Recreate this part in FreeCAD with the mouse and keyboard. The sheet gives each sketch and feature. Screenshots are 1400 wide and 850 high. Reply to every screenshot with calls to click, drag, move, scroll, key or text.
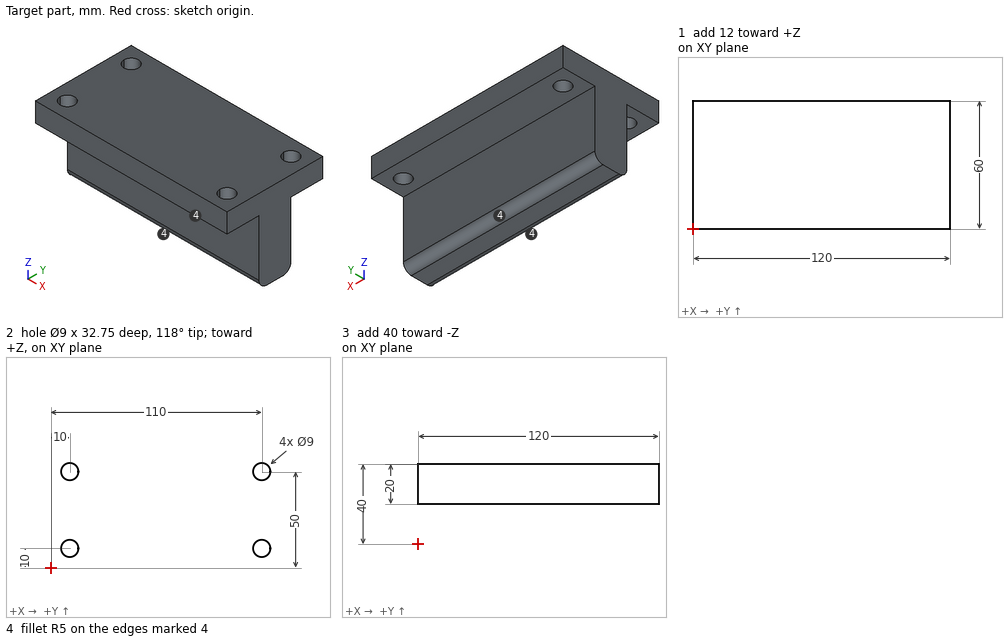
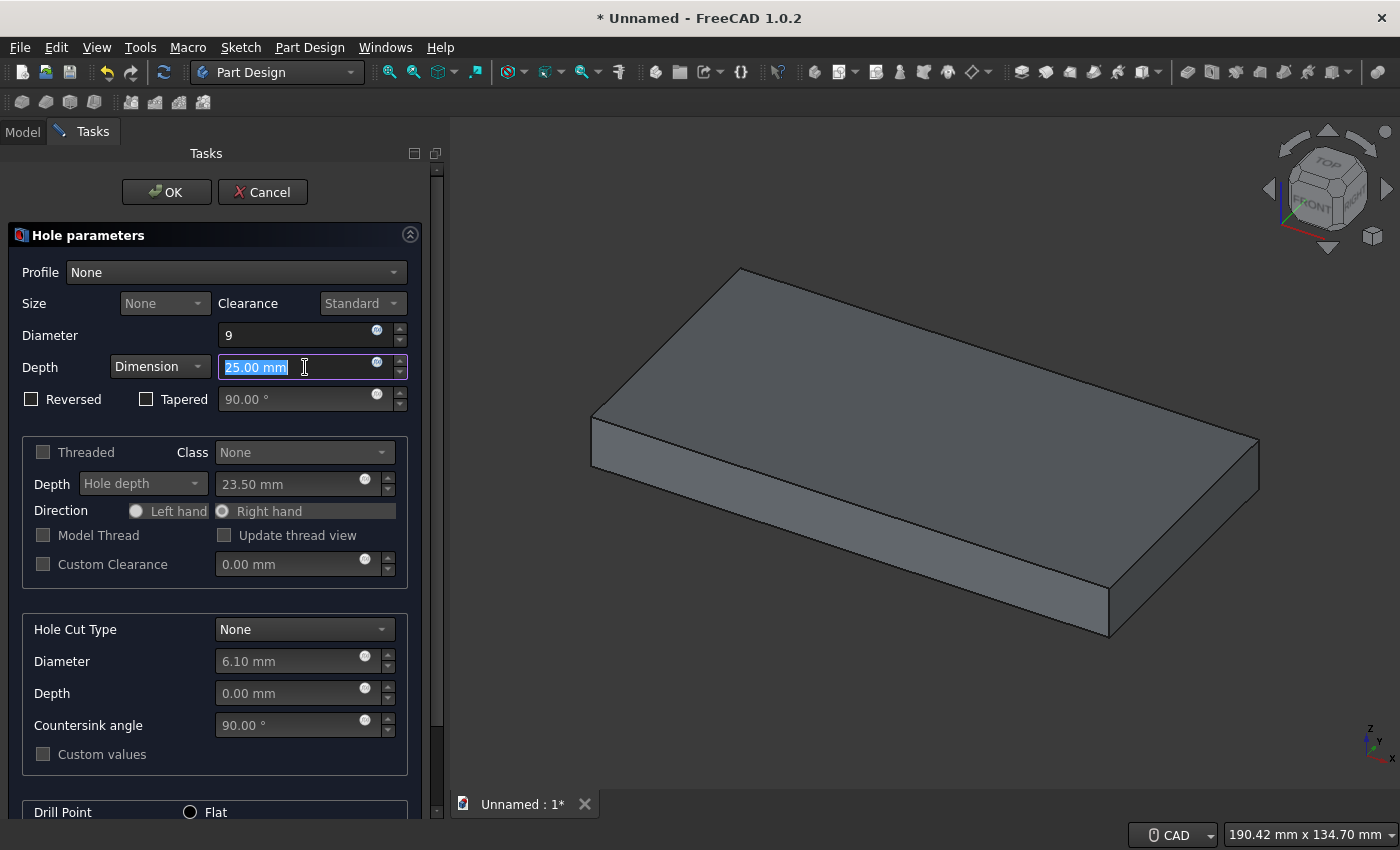
text(32.75)
key(Tab)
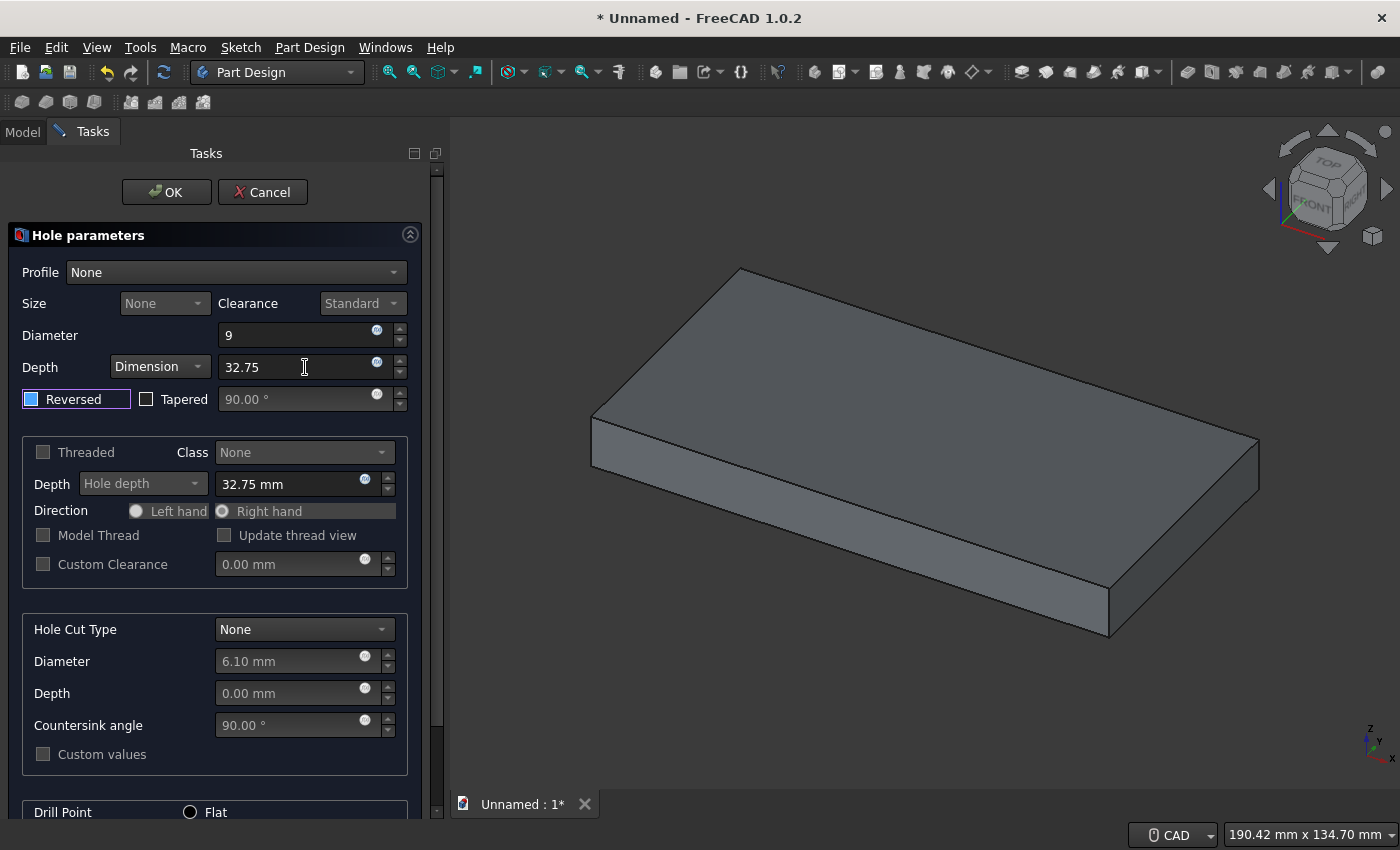
click(30, 399)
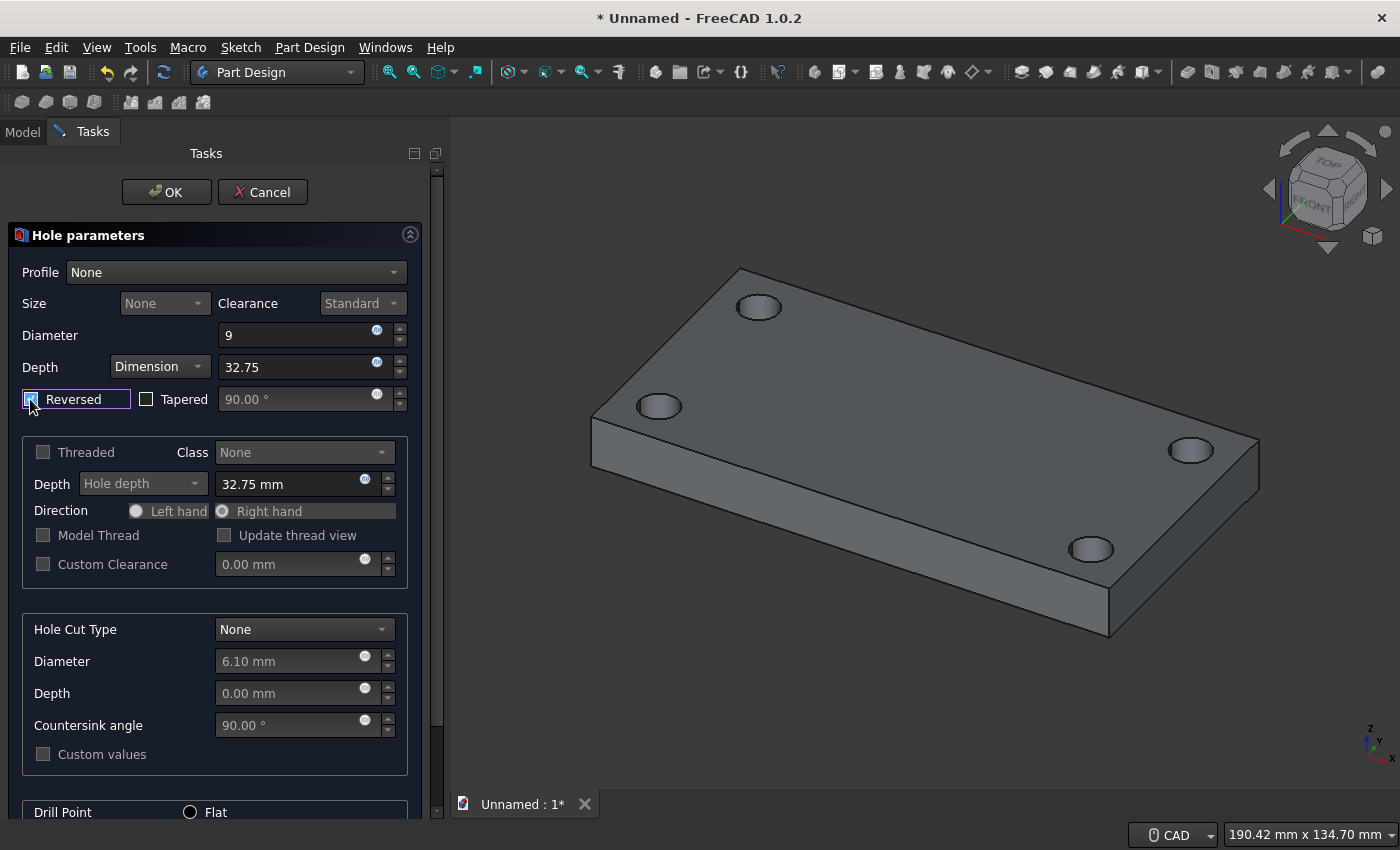
click(167, 192)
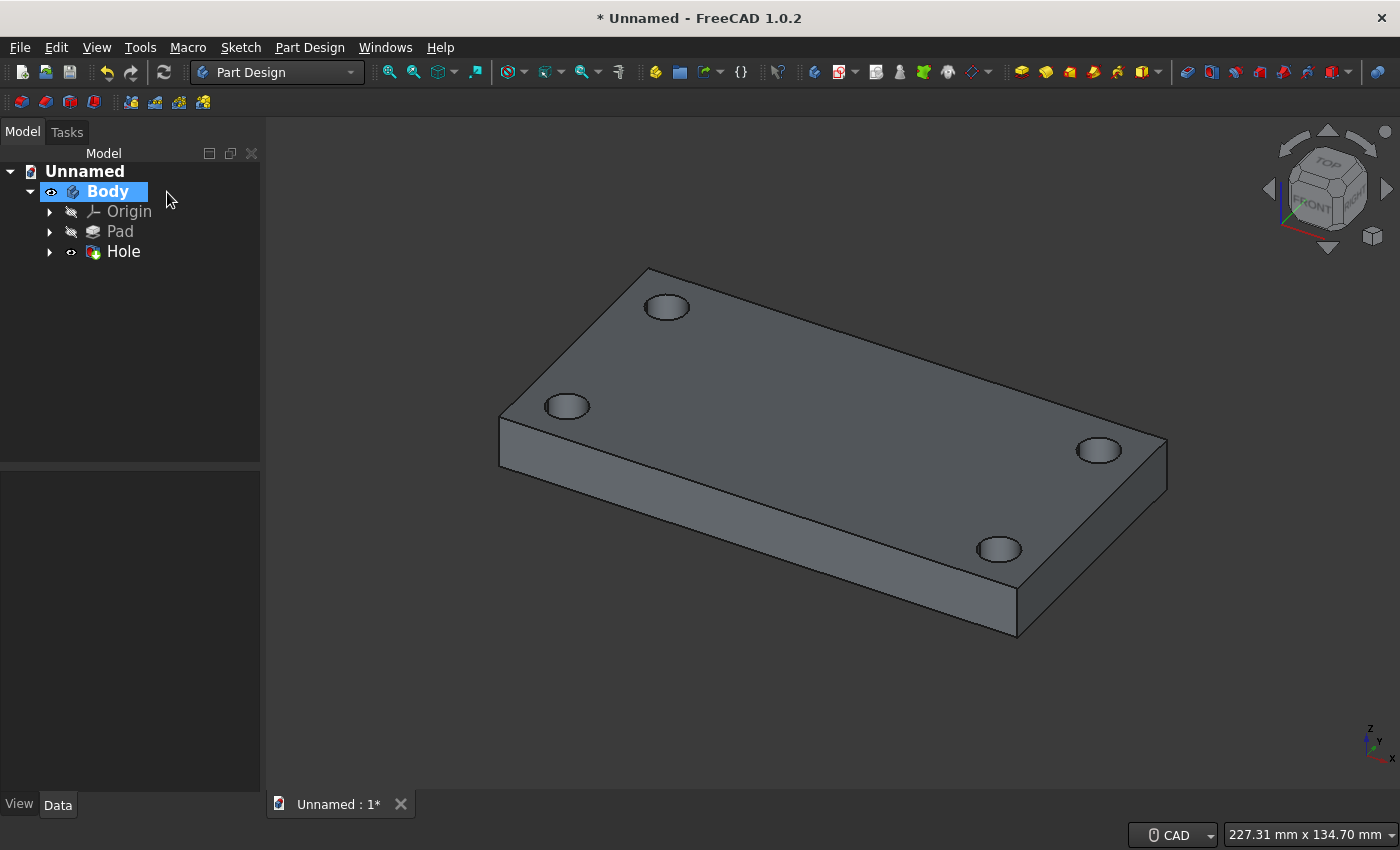
click(840, 72)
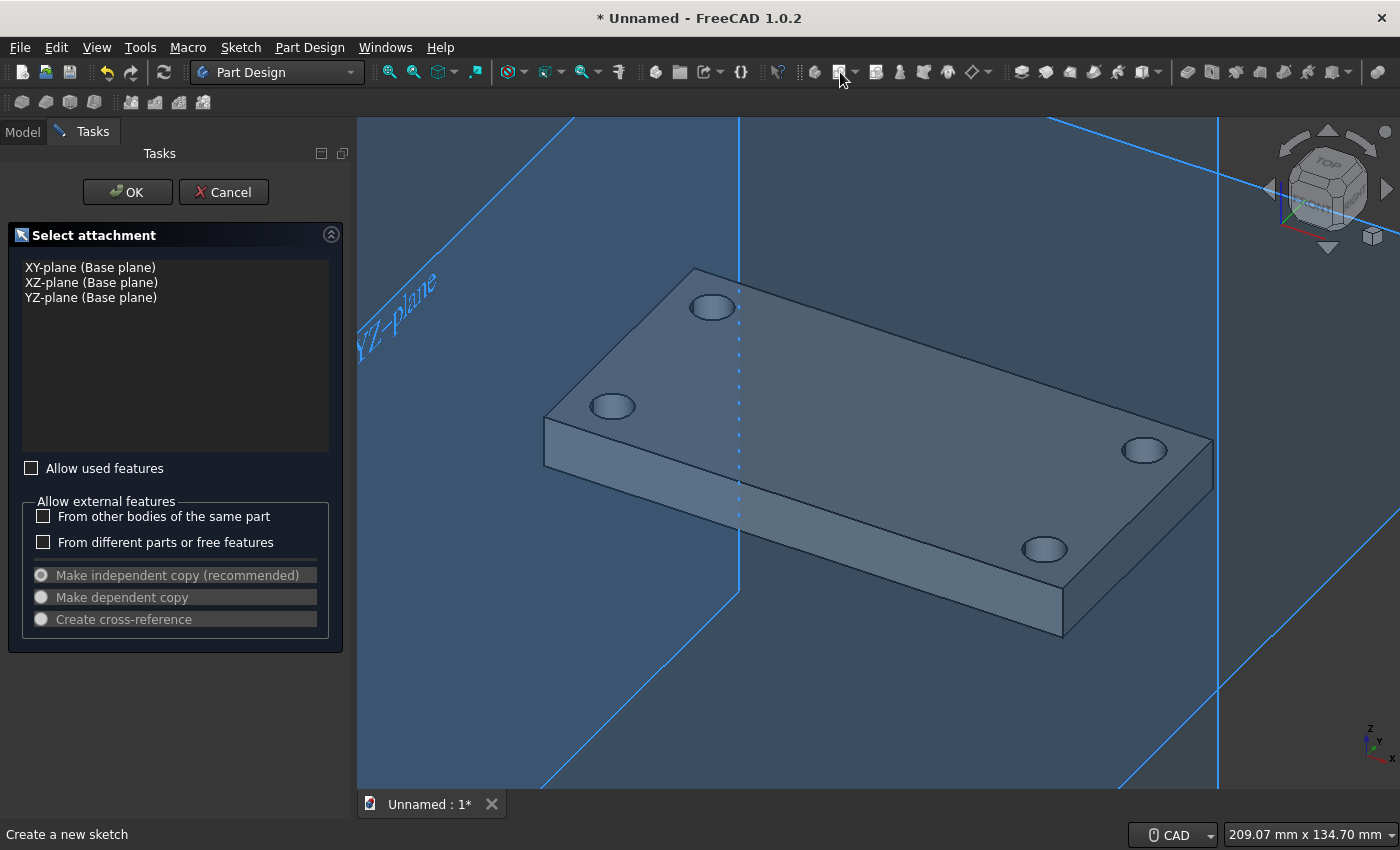
click(82, 268)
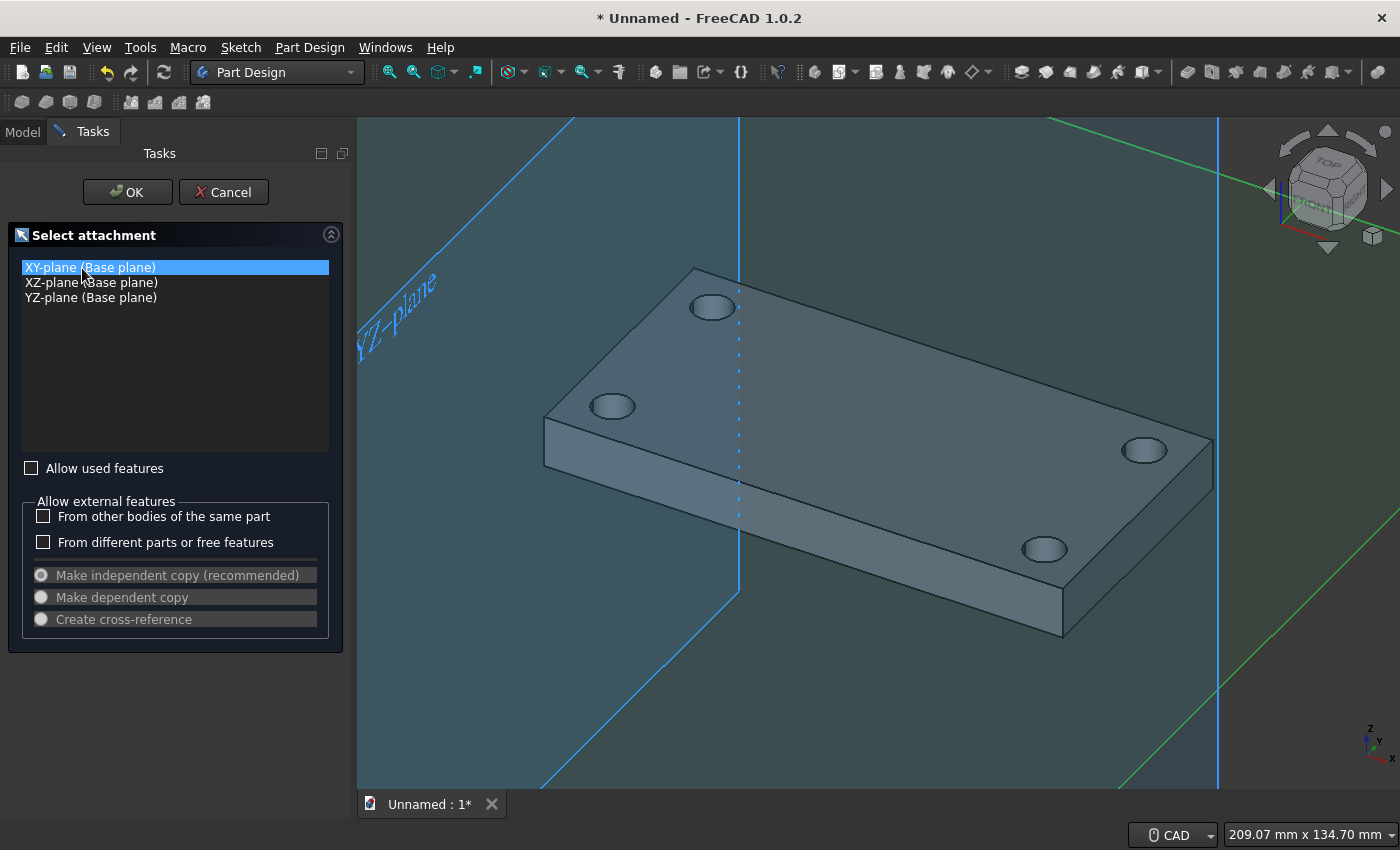
click(128, 192)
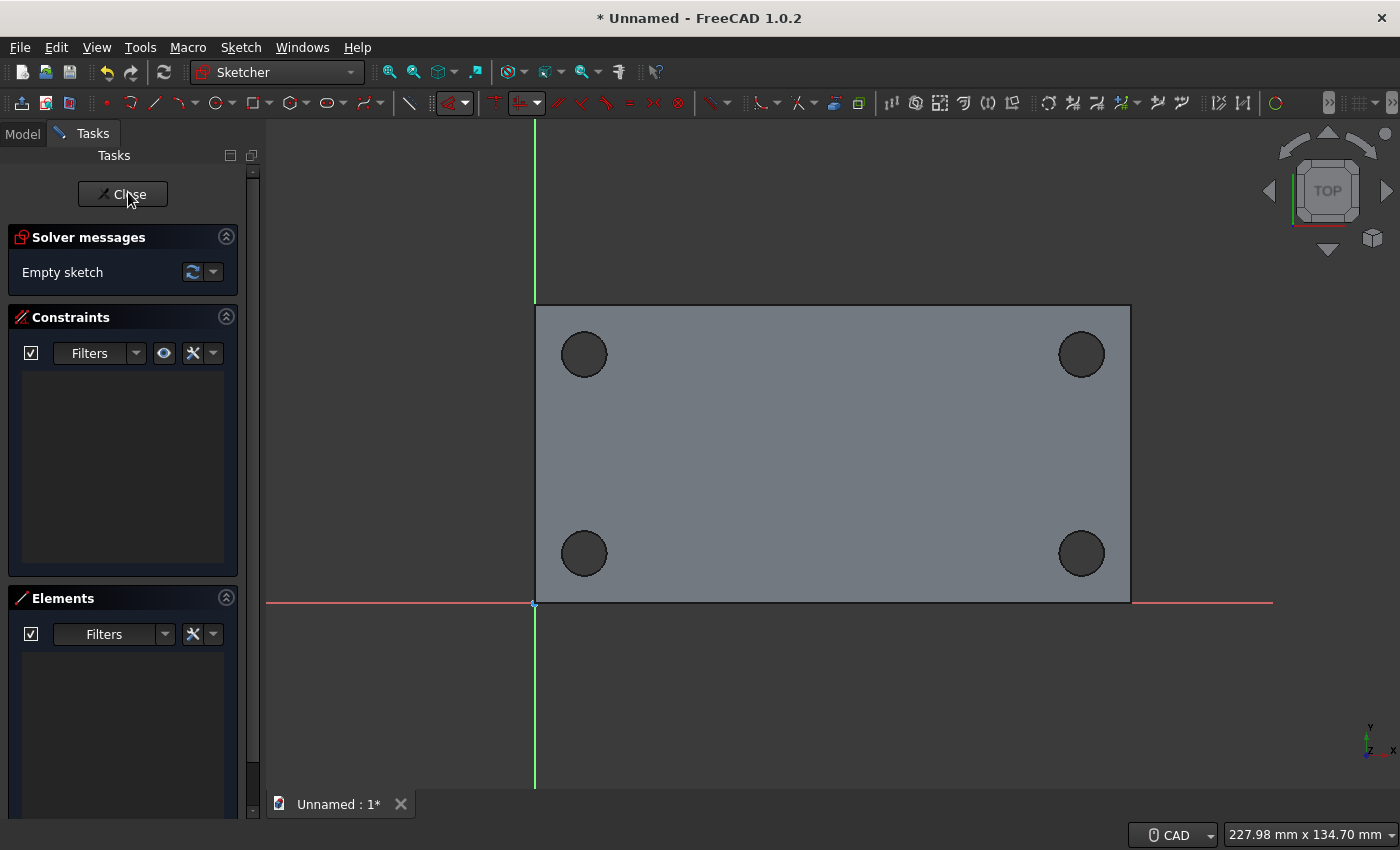
click(70, 104)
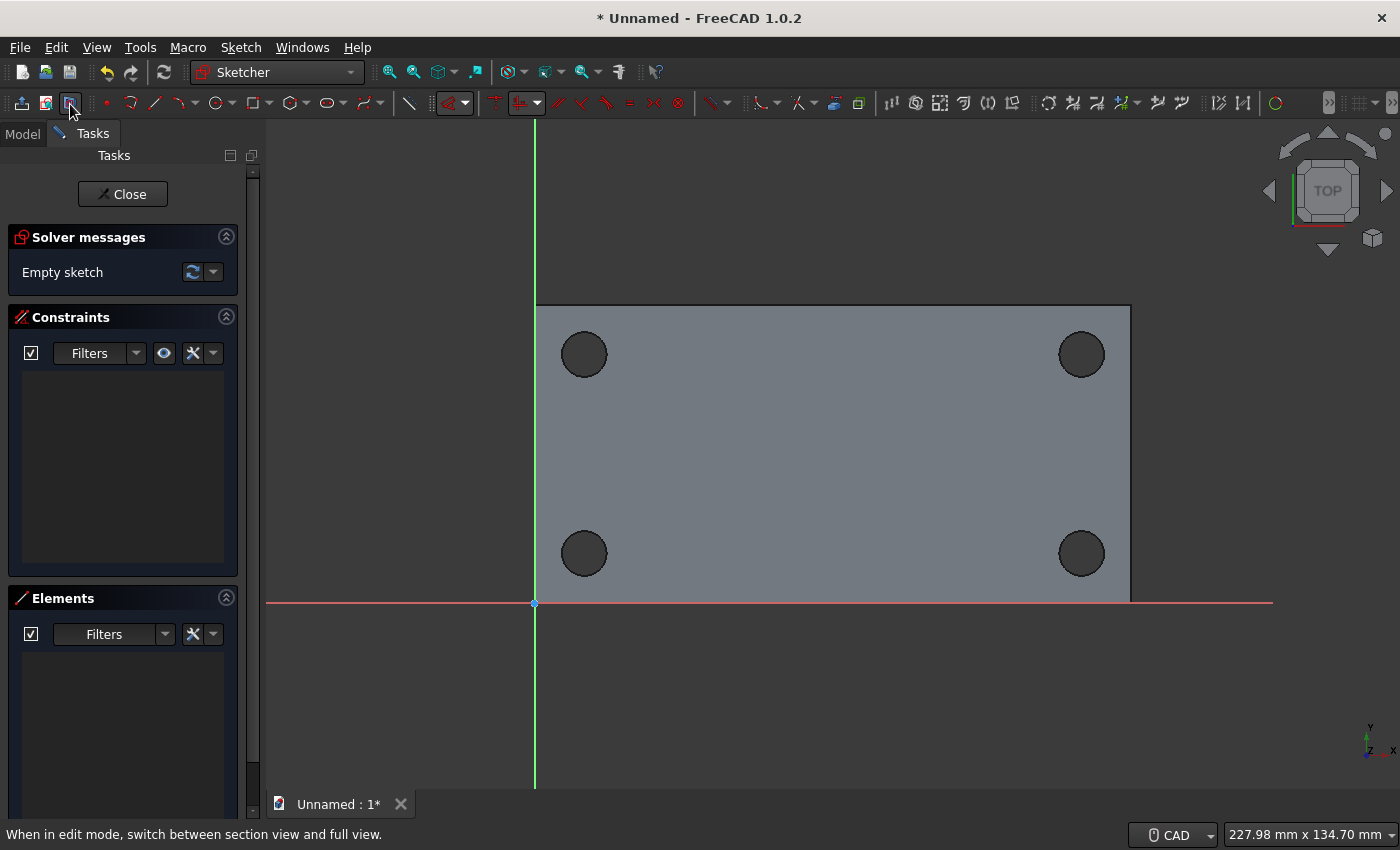
click(254, 104)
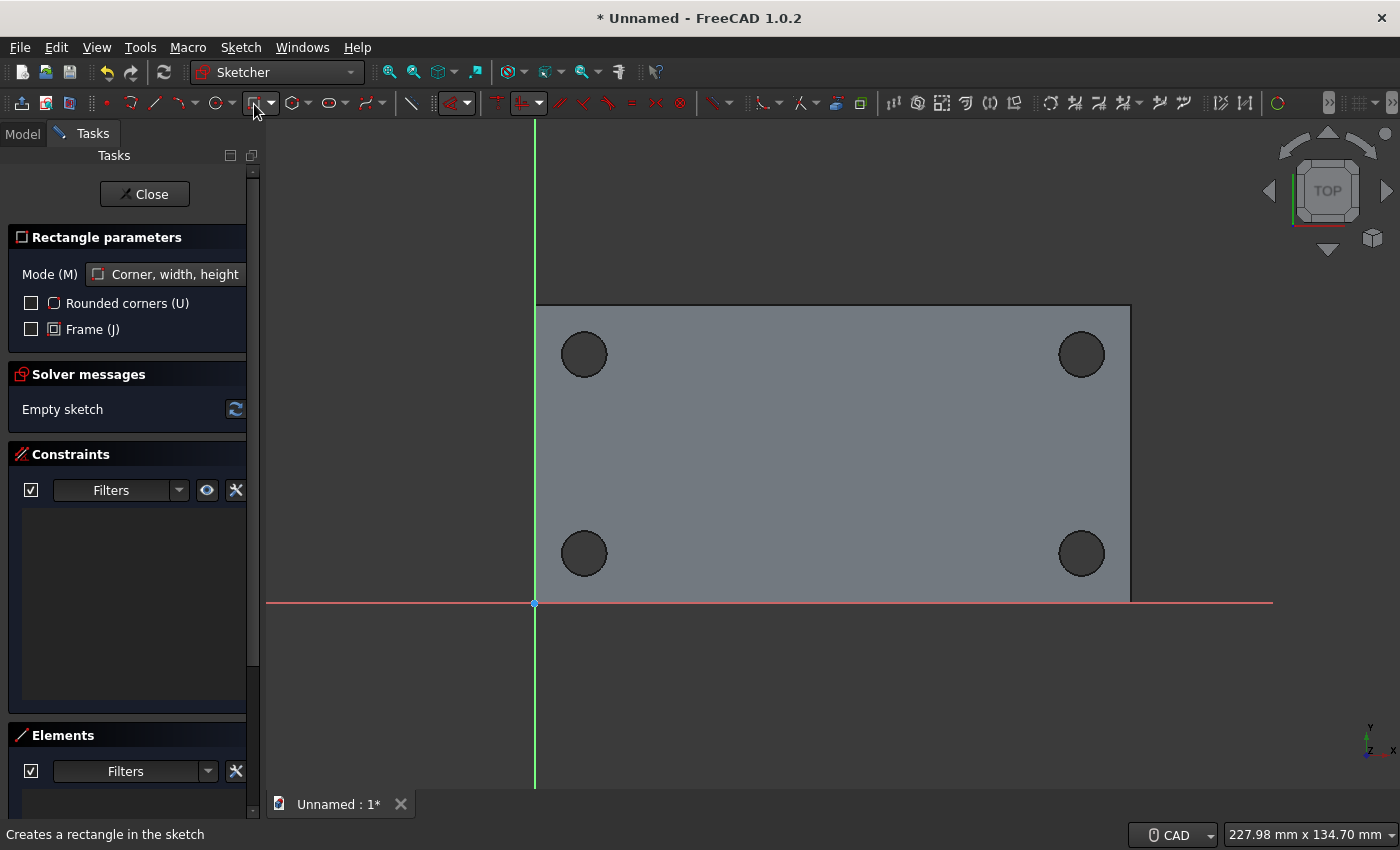
click(535, 404)
click(1131, 504)
key(Escape)